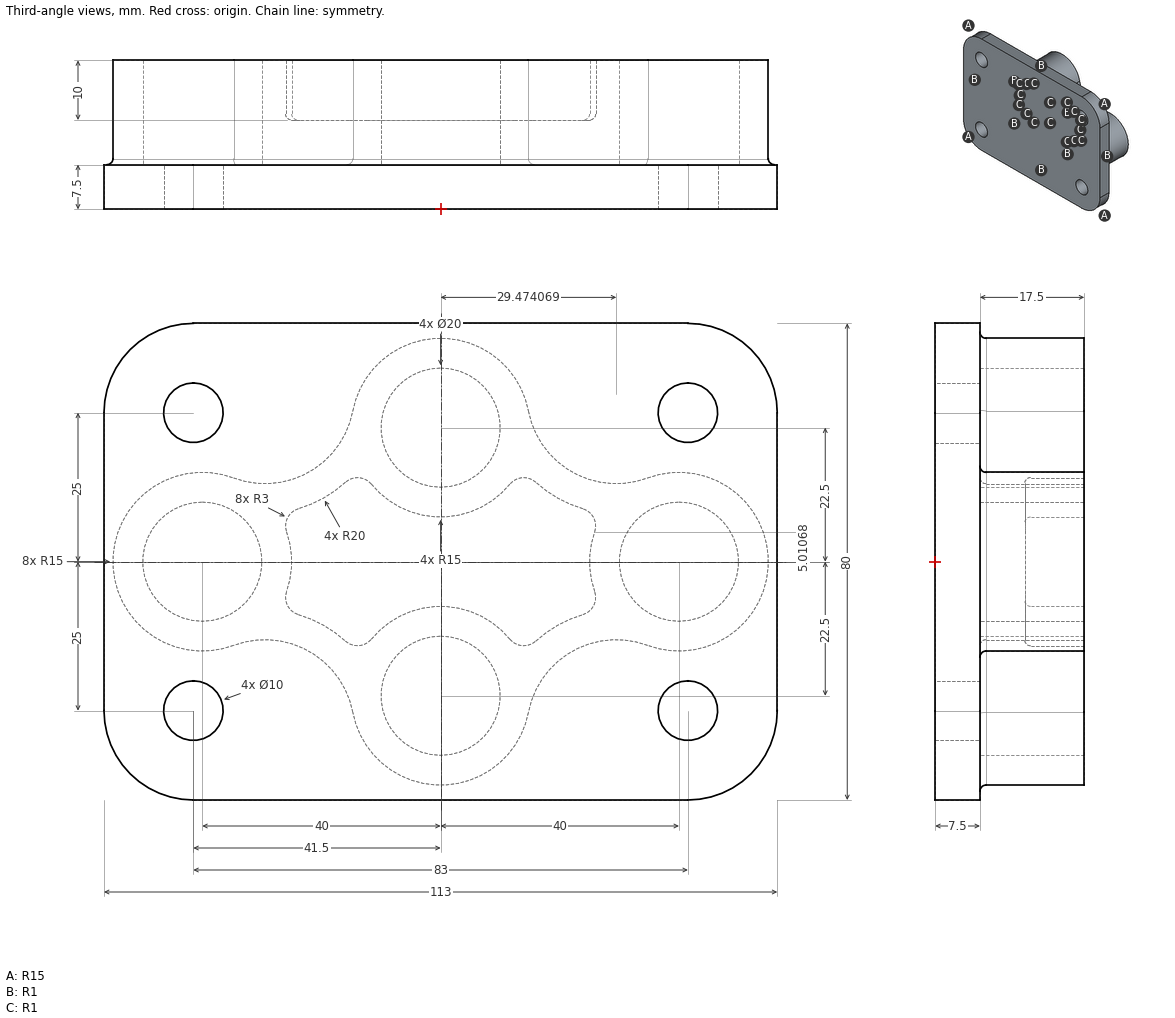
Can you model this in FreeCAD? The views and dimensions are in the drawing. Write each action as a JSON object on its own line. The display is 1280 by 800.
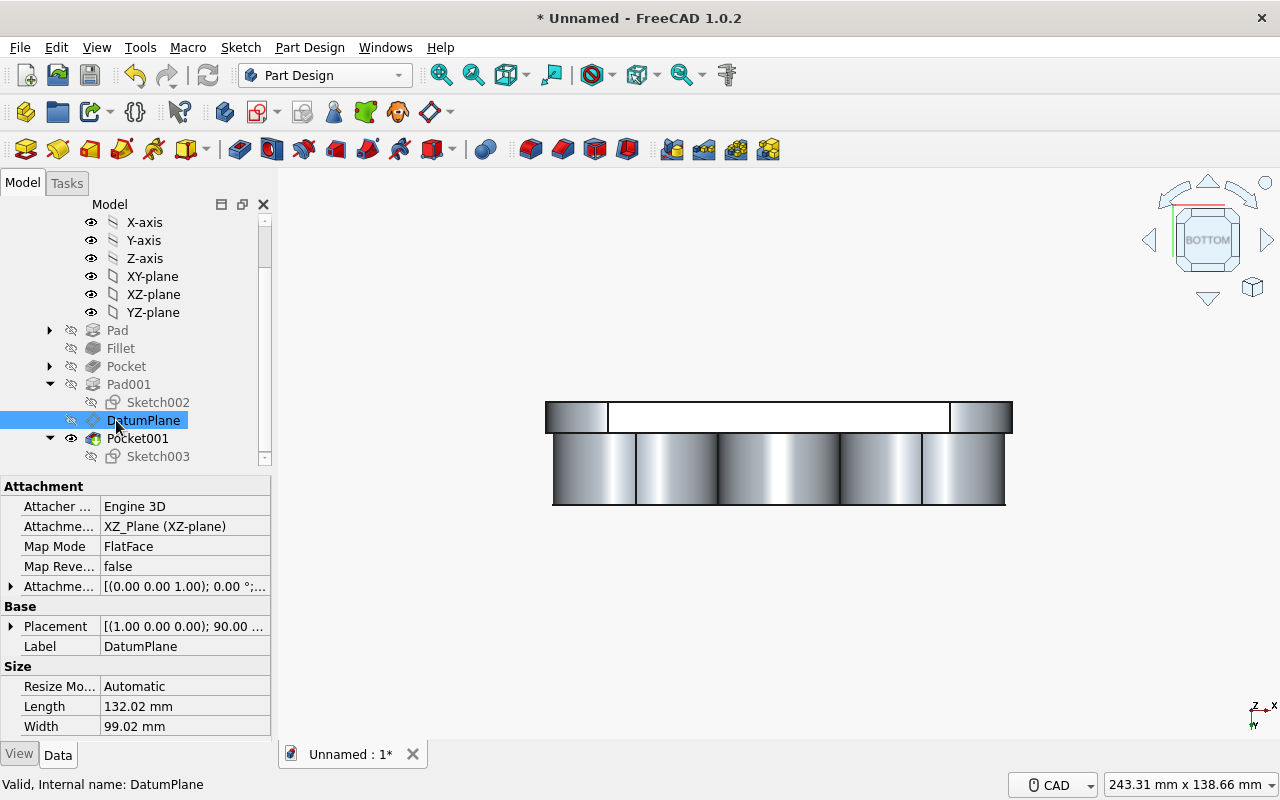
{"action": "key", "text": "4"}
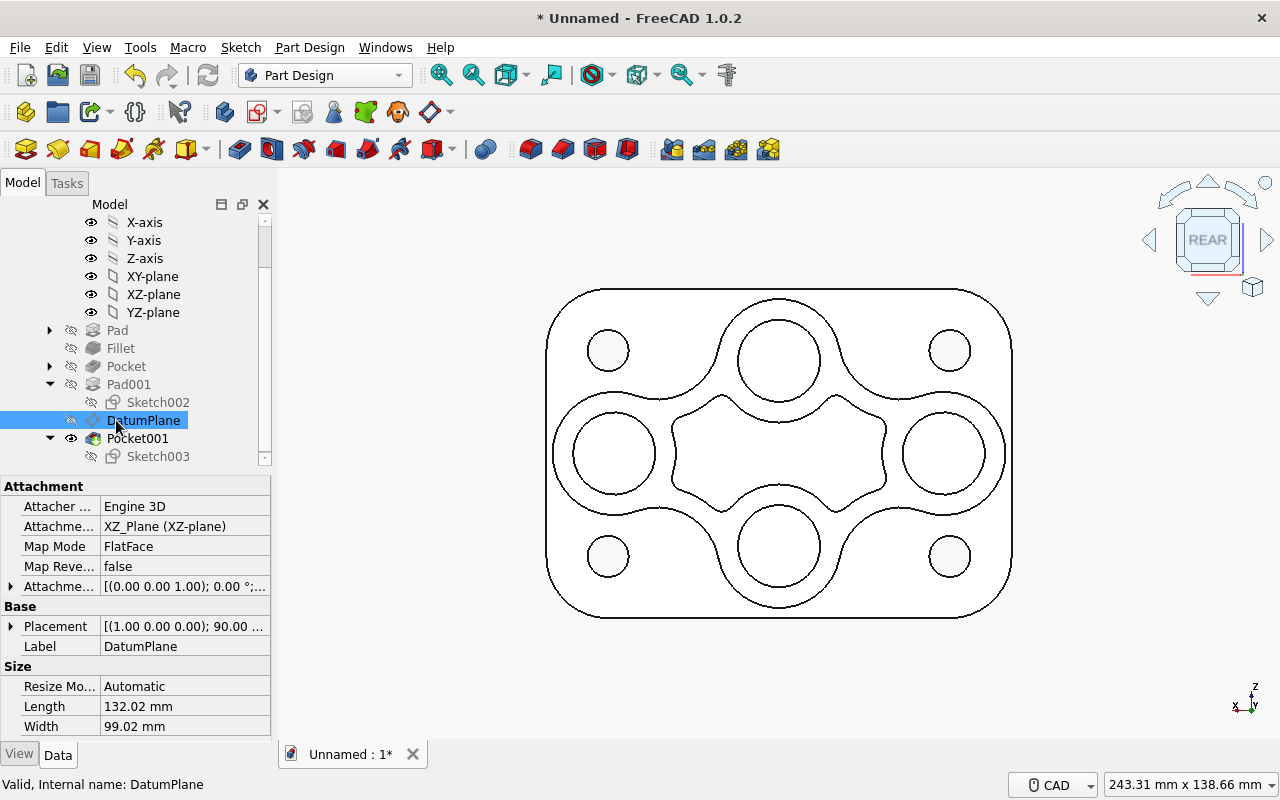
{"action": "key", "text": "6"}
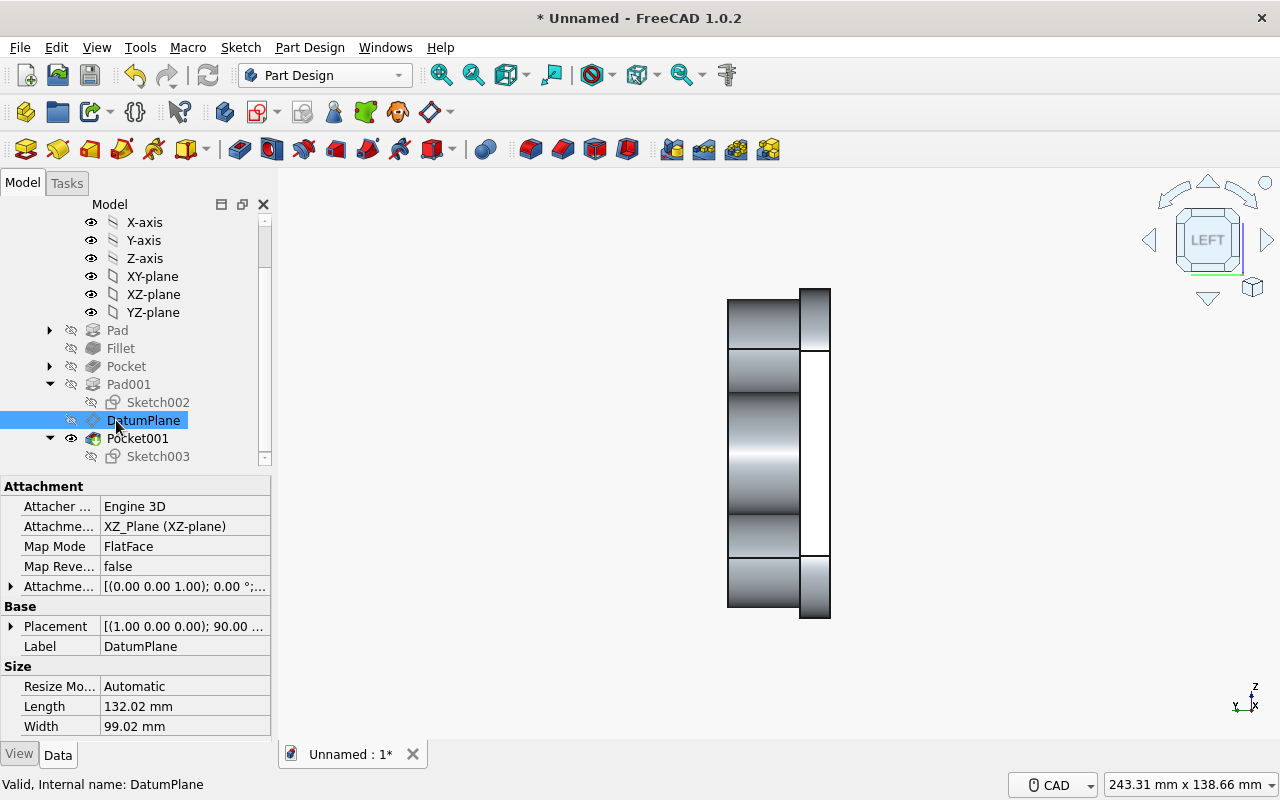
{"action": "key", "text": "v 3"}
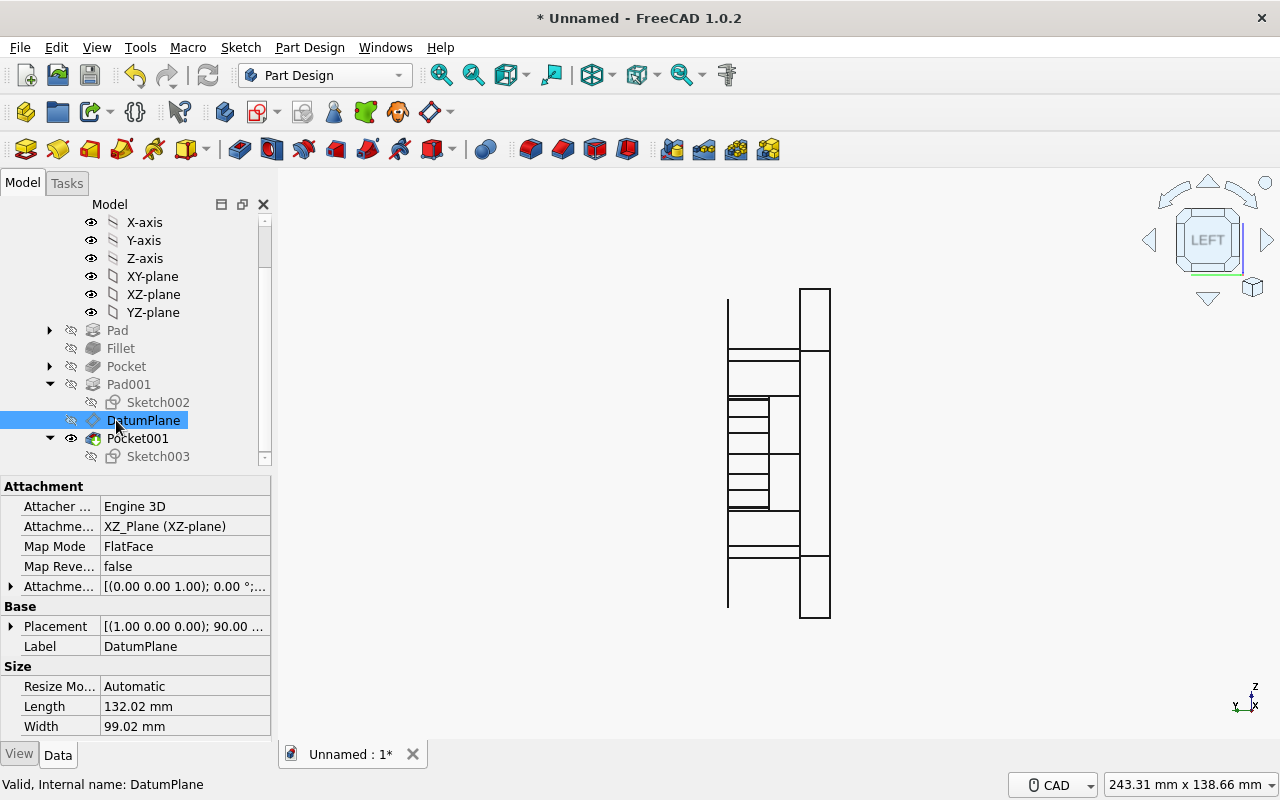
{"action": "key", "text": "0"}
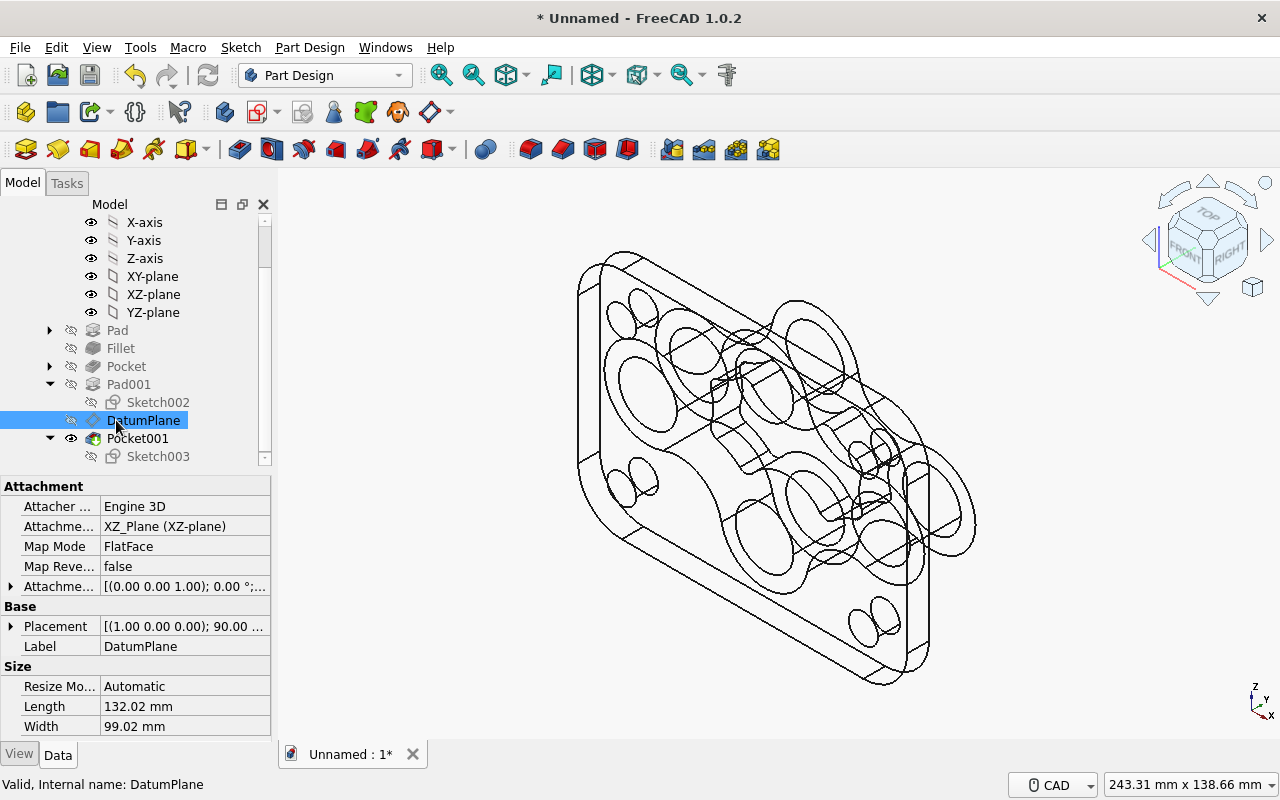
{"action": "left_click", "coordinate": [700, 474]}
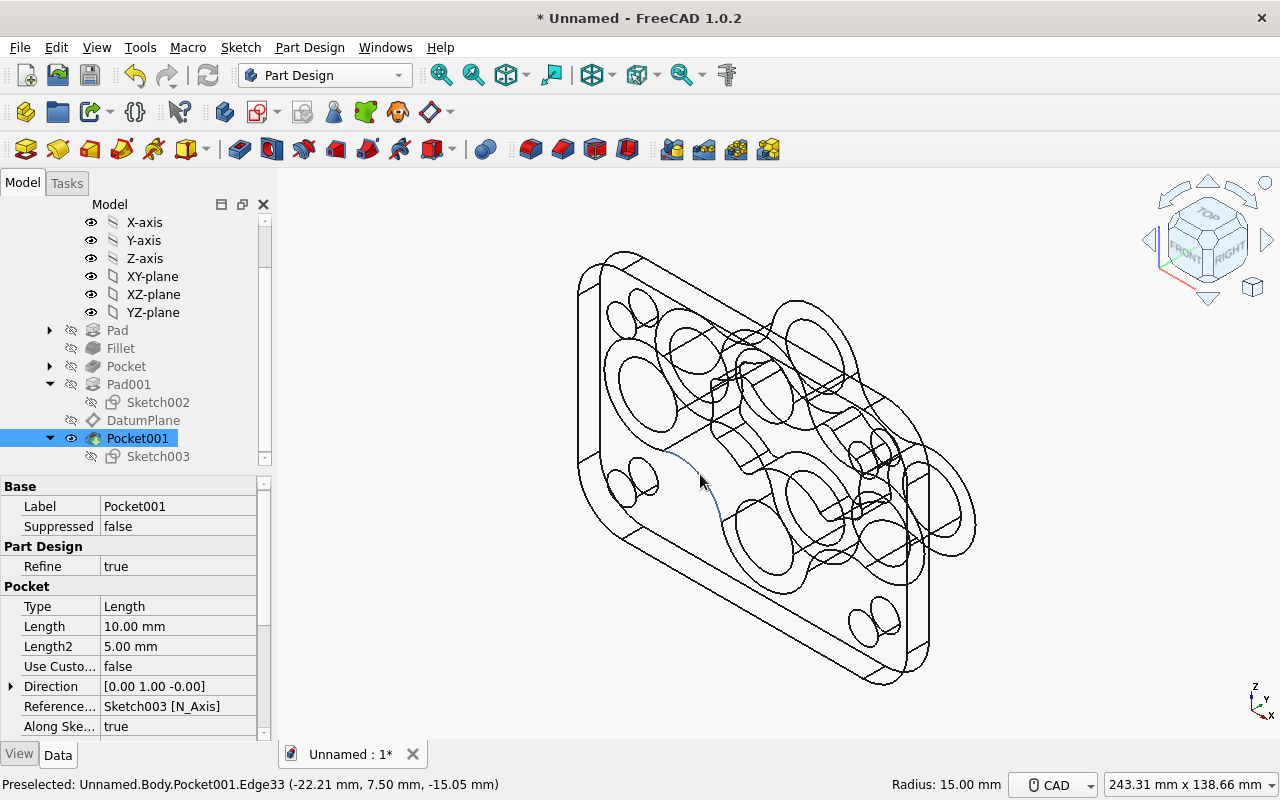
{"action": "left_click", "coordinate": [604, 368], "text": "ctrl"}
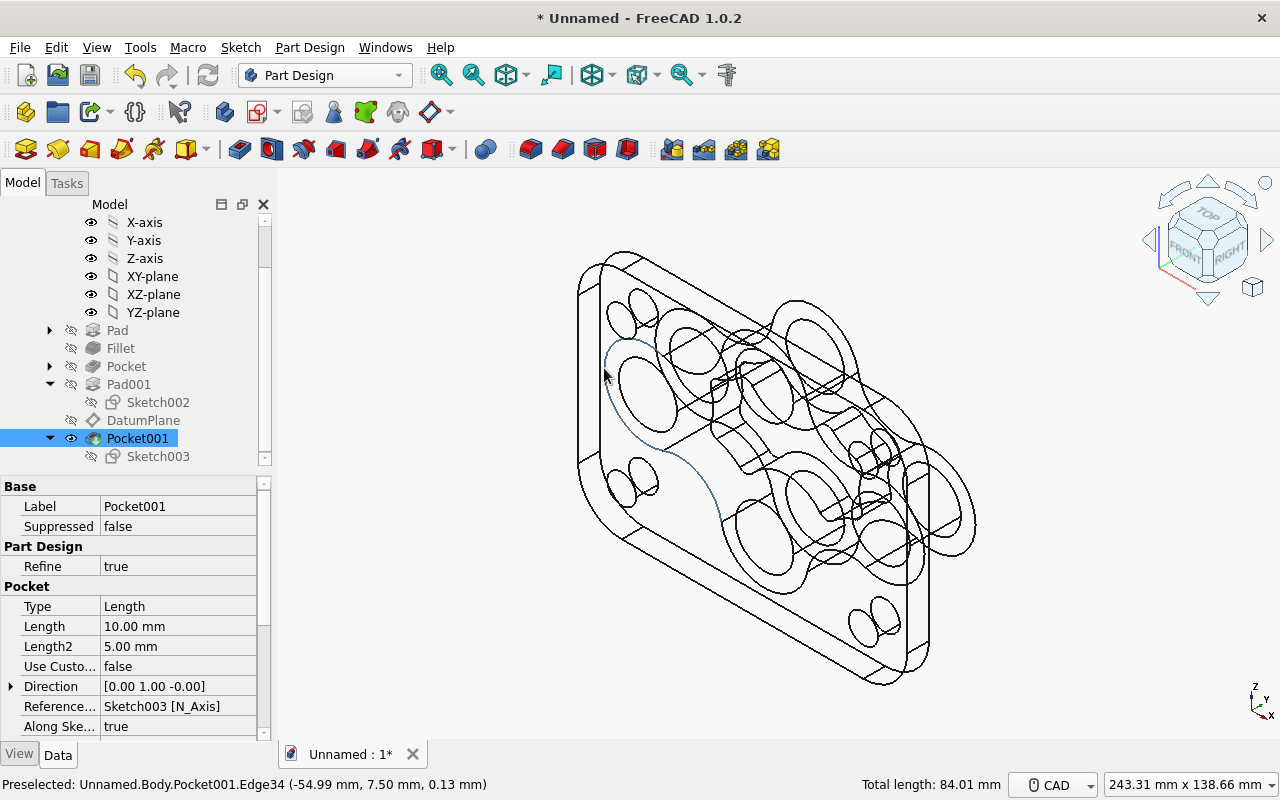
{"action": "left_click", "coordinate": [700, 373], "text": "ctrl"}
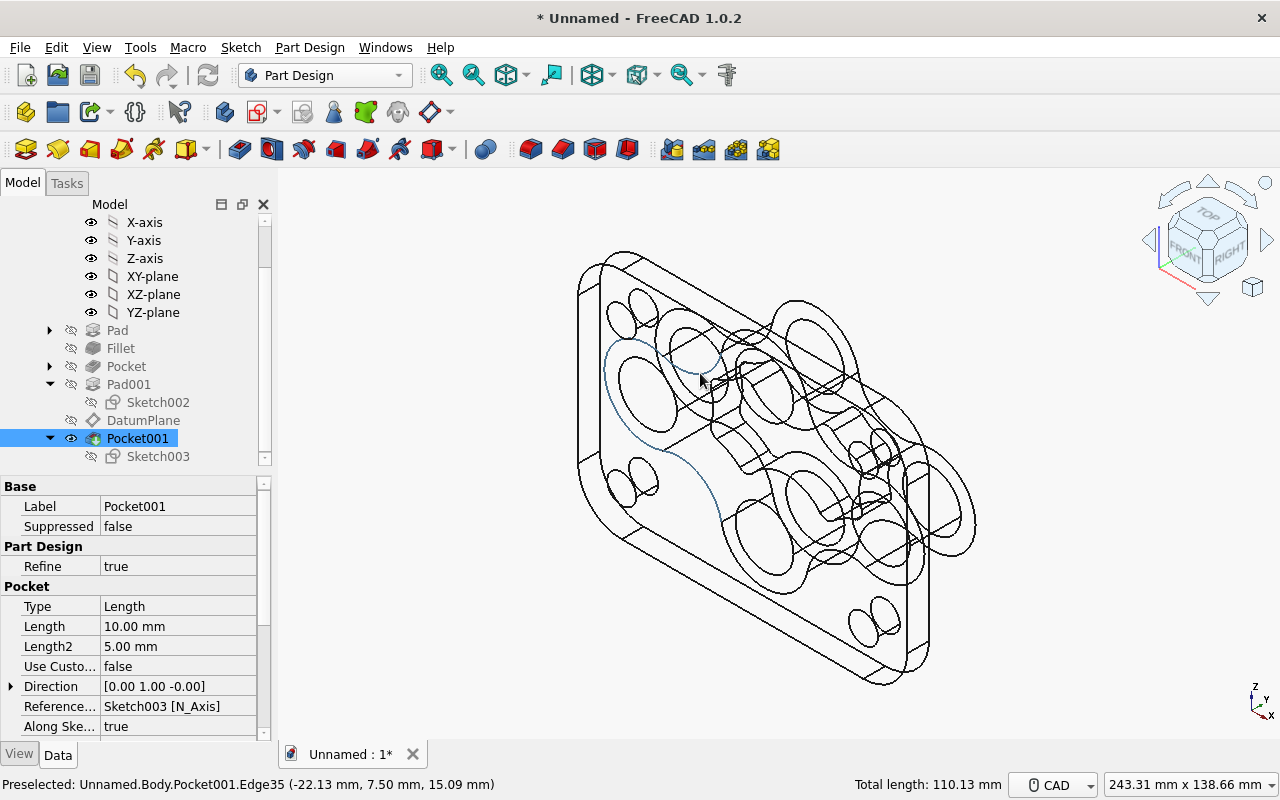
{"action": "left_click", "coordinate": [764, 335], "text": "ctrl"}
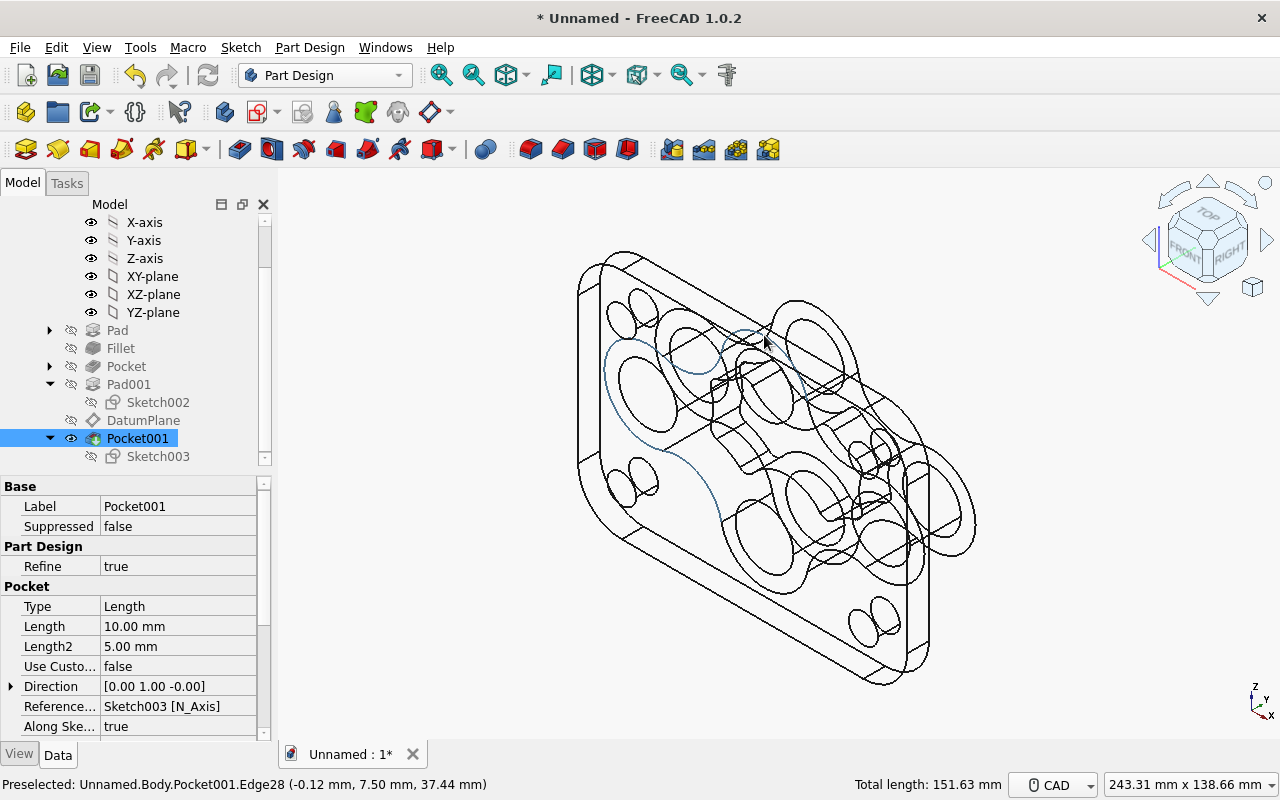
{"action": "left_click", "coordinate": [829, 448], "text": "ctrl"}